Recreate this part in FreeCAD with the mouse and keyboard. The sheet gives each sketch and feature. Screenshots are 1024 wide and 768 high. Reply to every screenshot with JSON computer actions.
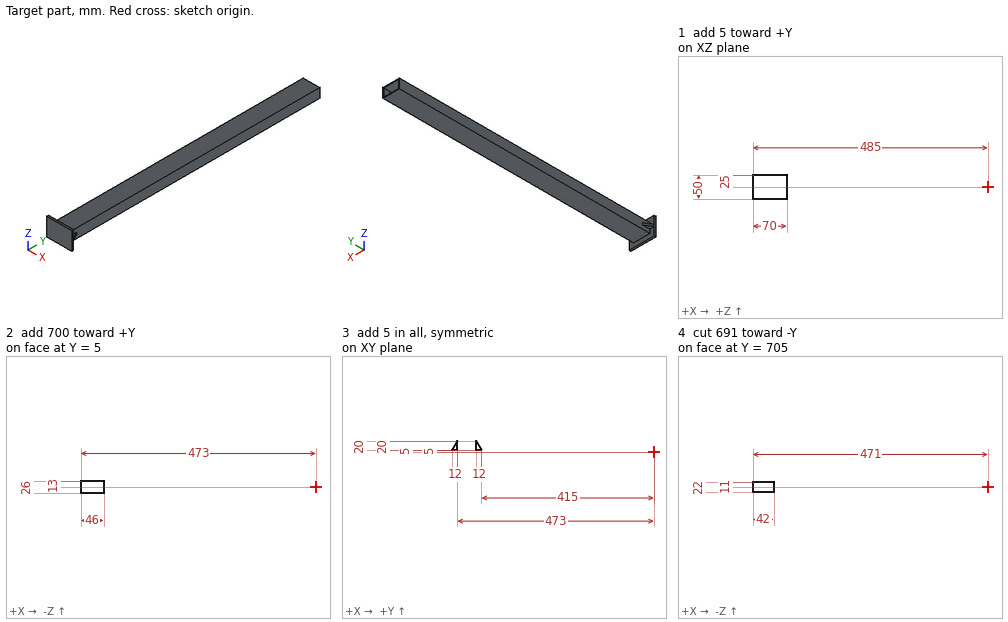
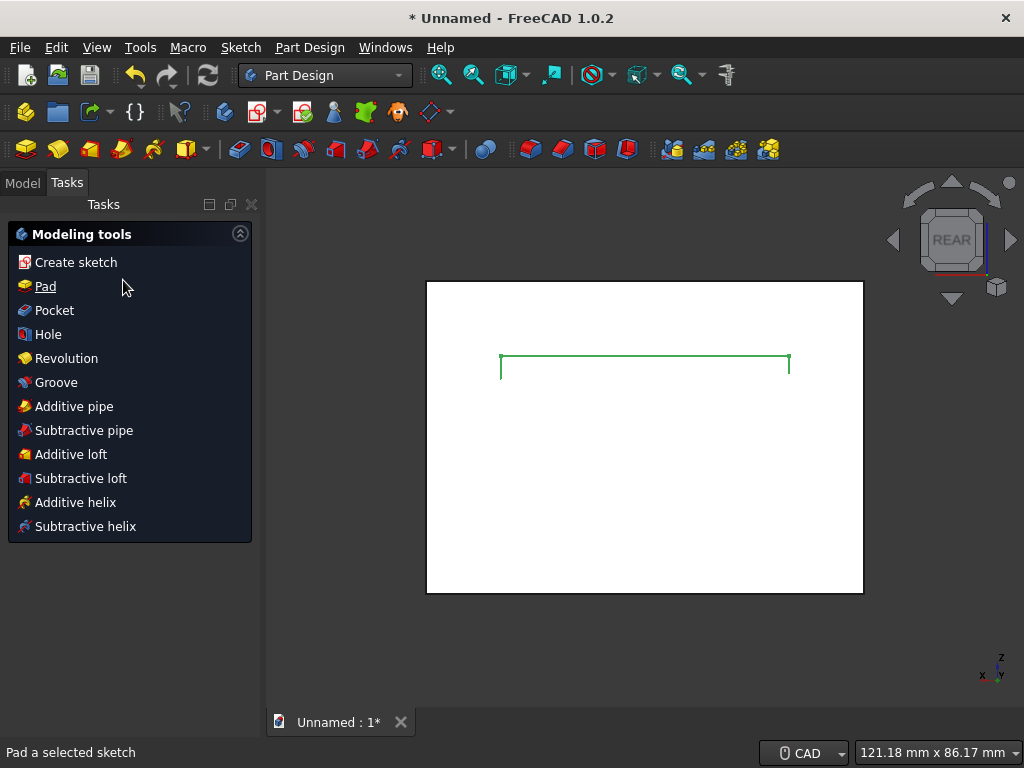
{"action": "left_click", "coordinate": [26, 150]}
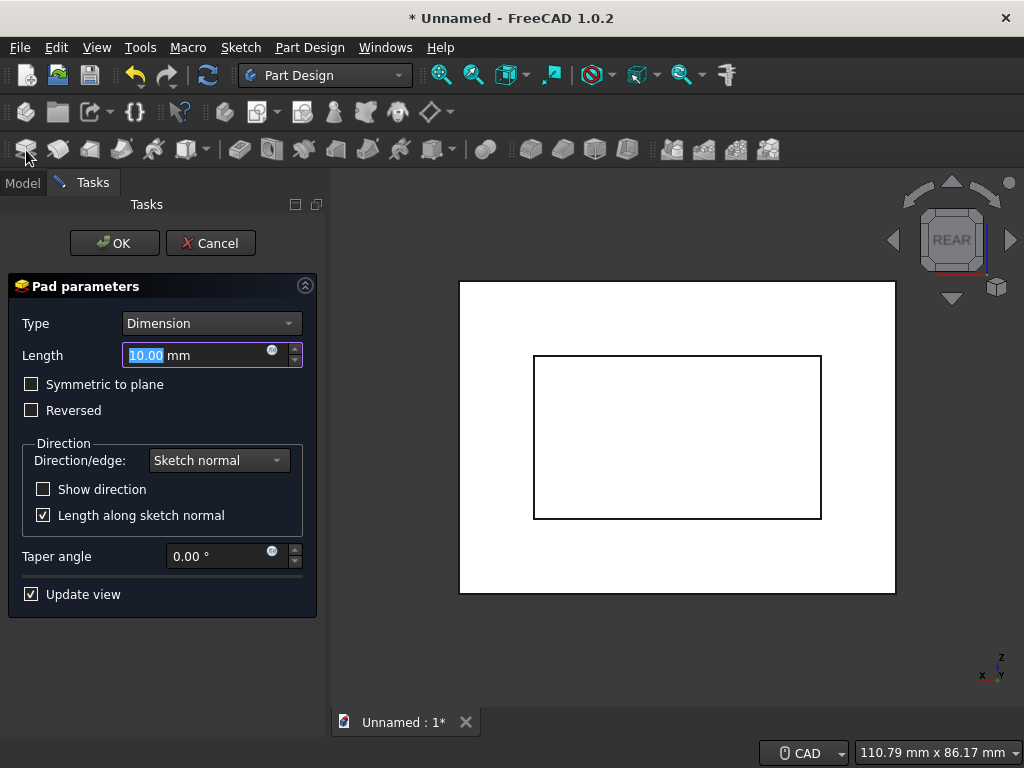
{"action": "type", "text": "700"}
{"action": "key", "text": "Tab"}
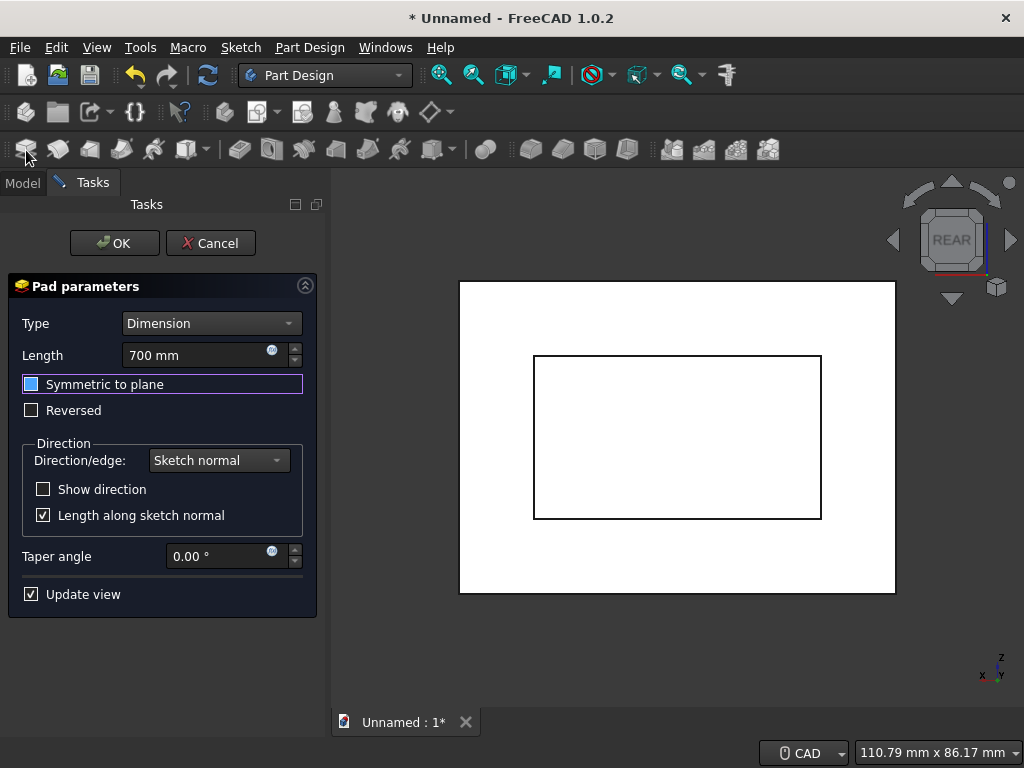
{"action": "left_click", "coordinate": [115, 243]}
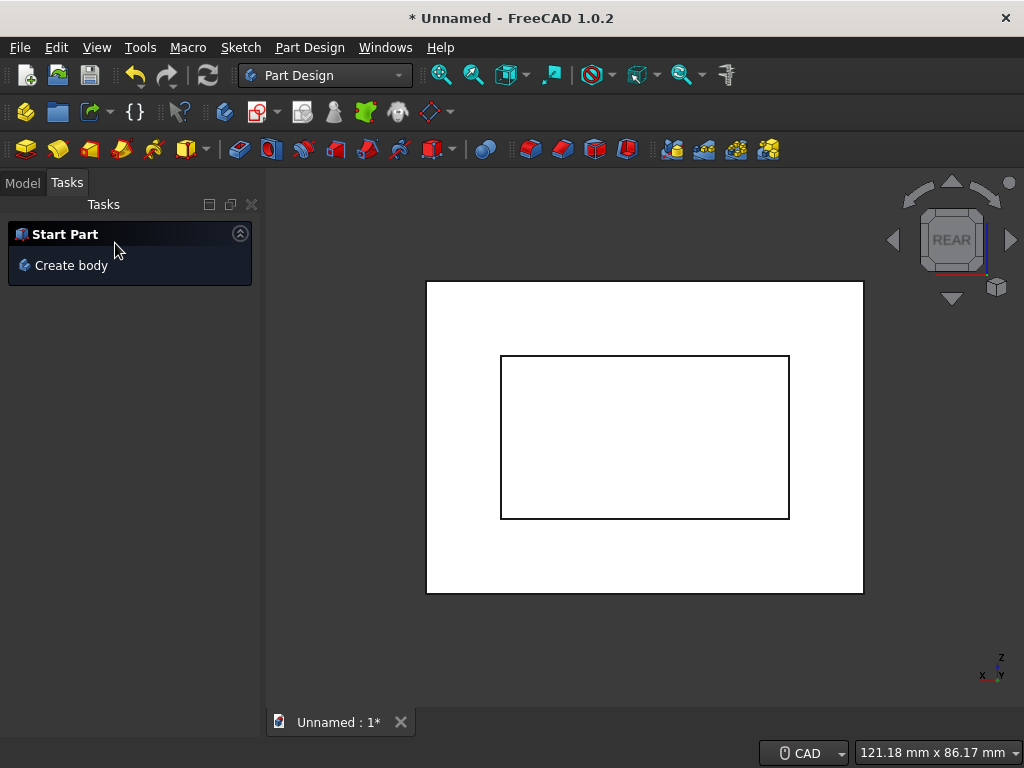
{"action": "left_click", "coordinate": [258, 112]}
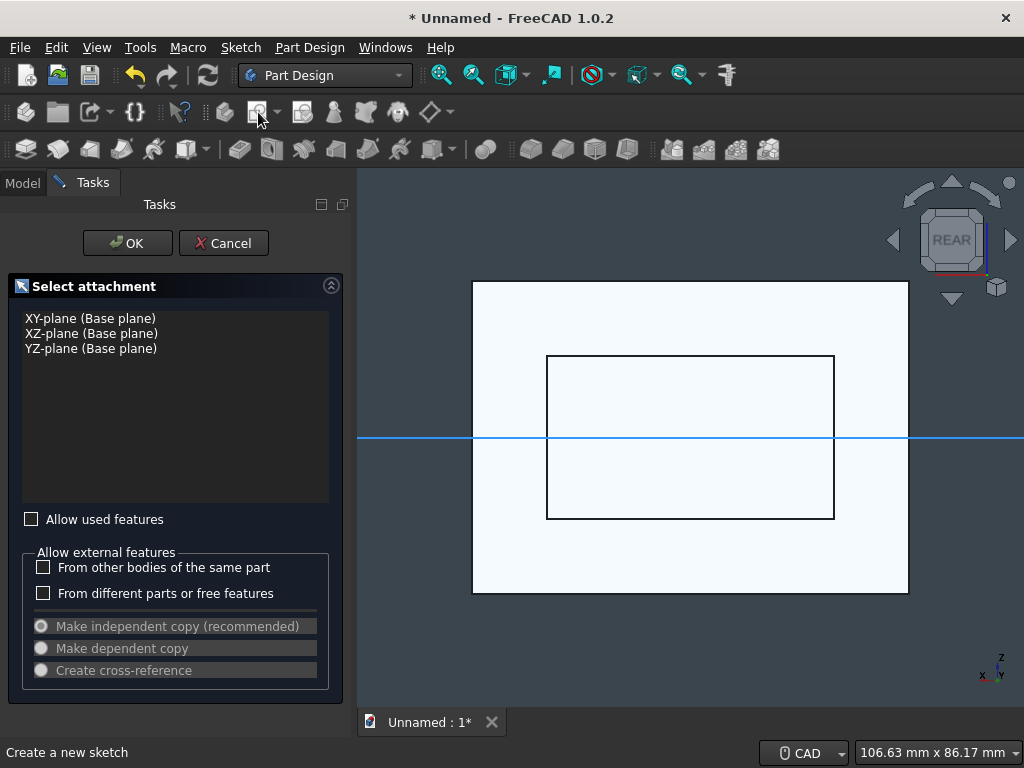
{"action": "left_click", "coordinate": [82, 318]}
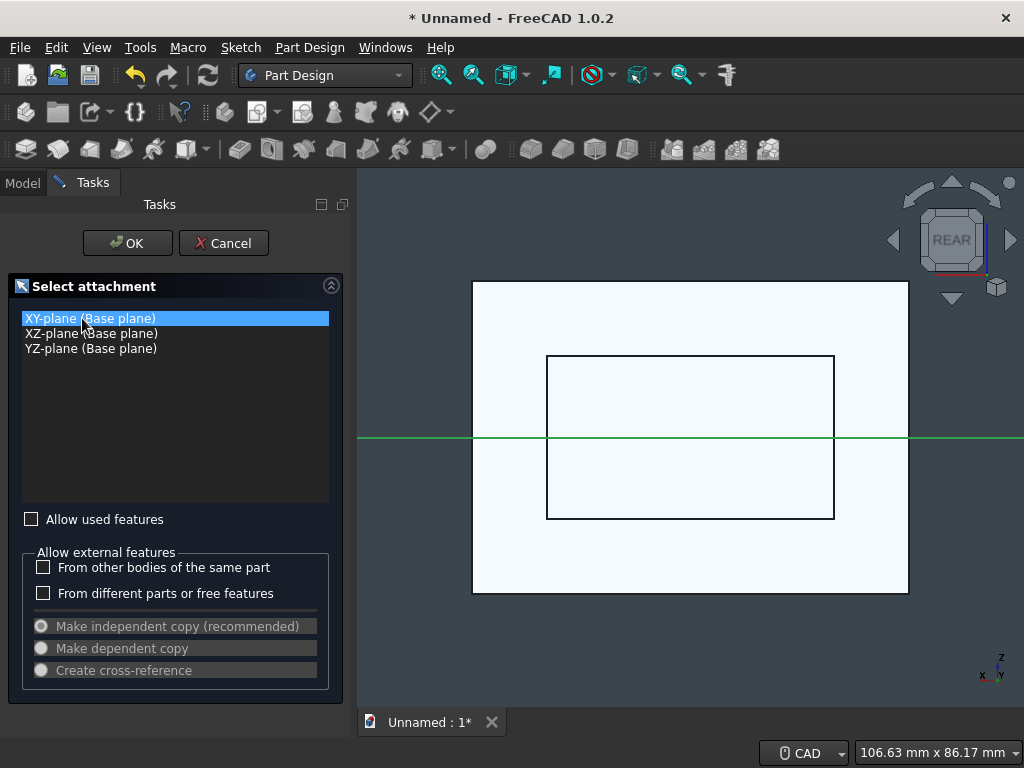
{"action": "left_click", "coordinate": [128, 243]}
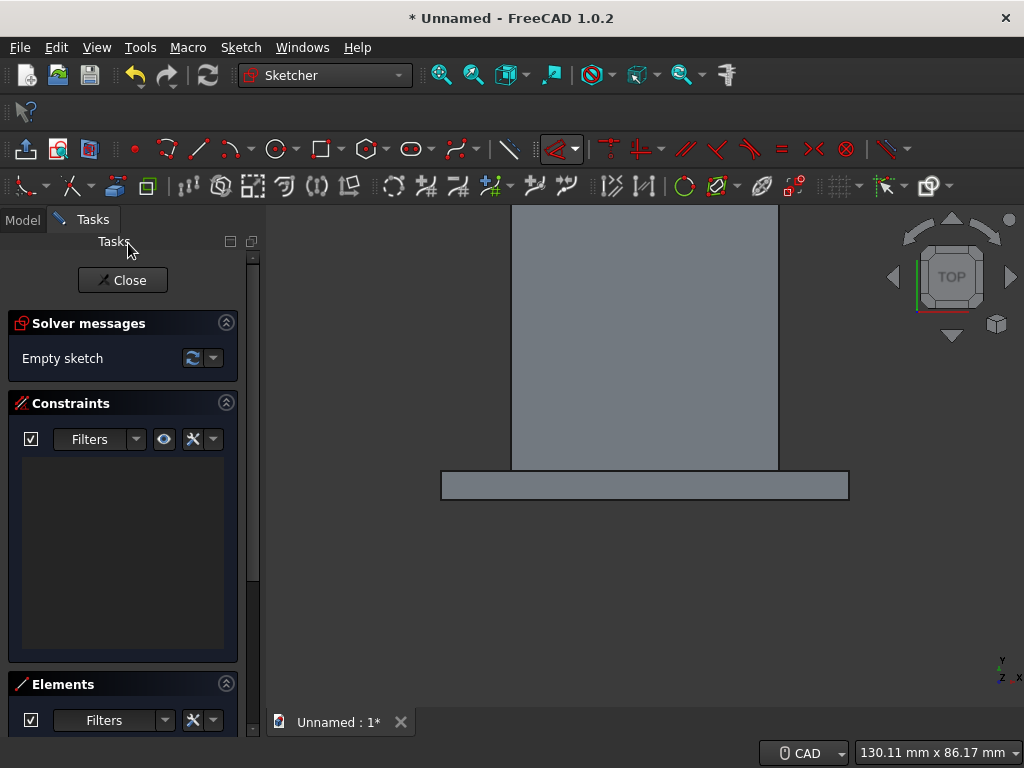
{"action": "left_click", "coordinate": [90, 150]}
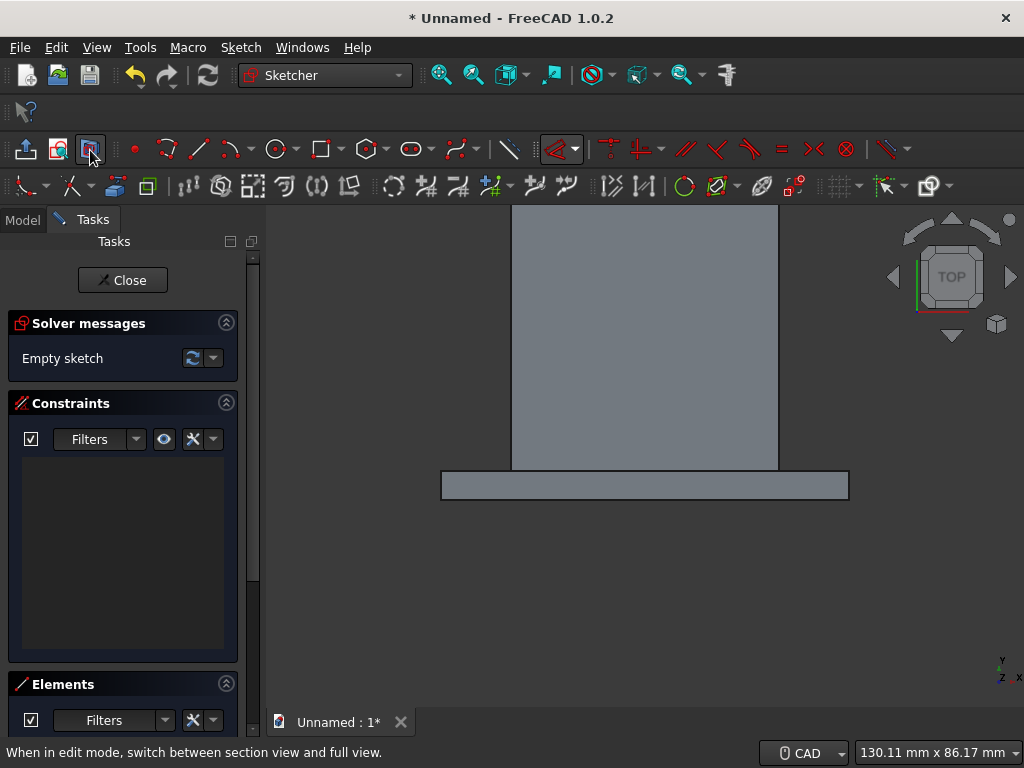
{"action": "scroll", "coordinate": [294, 653], "scroll_direction": "down", "scroll_amount": 1}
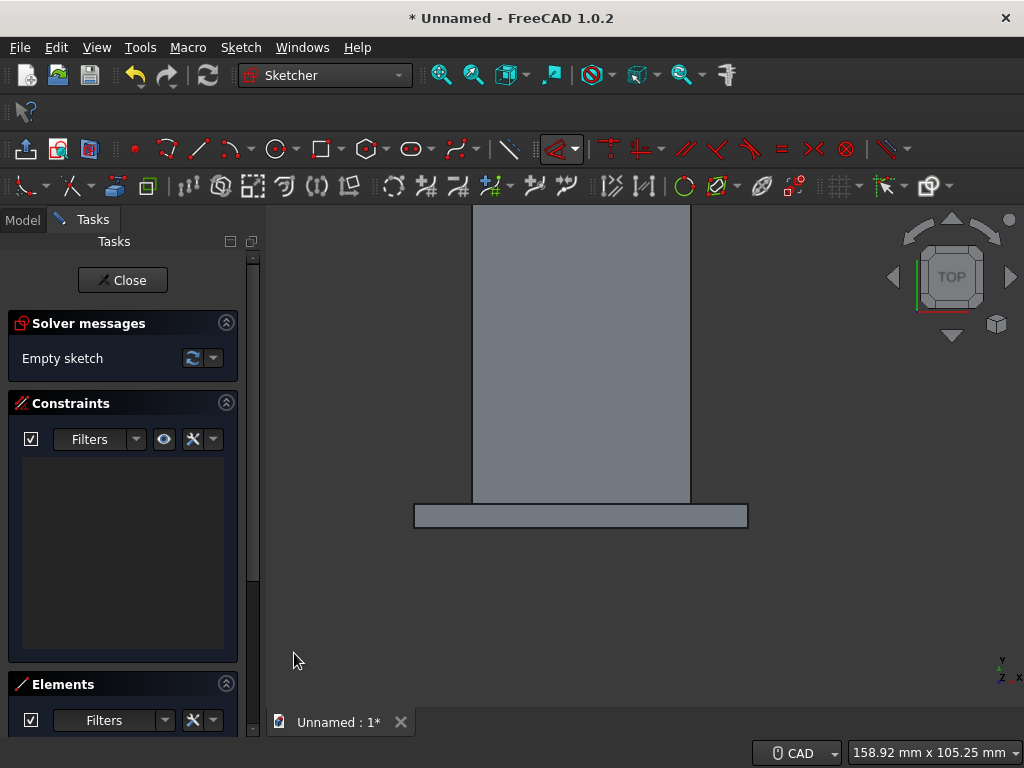
{"action": "left_click", "coordinate": [168, 150]}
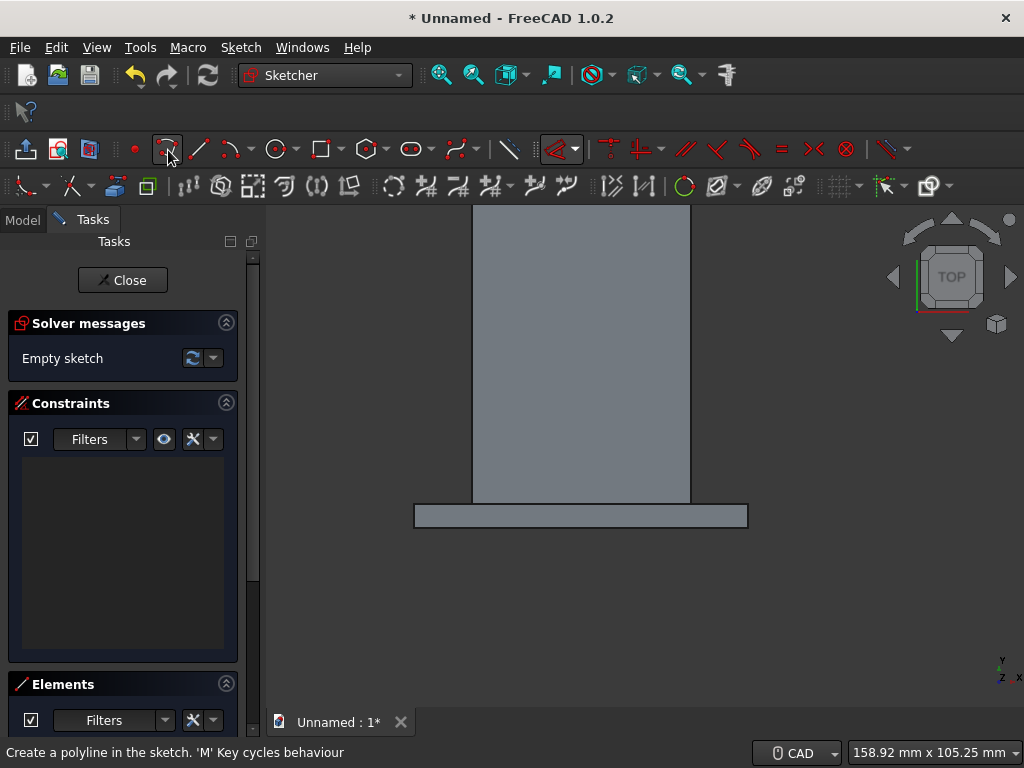
{"action": "left_click", "coordinate": [472, 504]}
{"action": "left_click", "coordinate": [472, 408]}
{"action": "left_click", "coordinate": [414, 504]}
{"action": "left_click", "coordinate": [472, 505]}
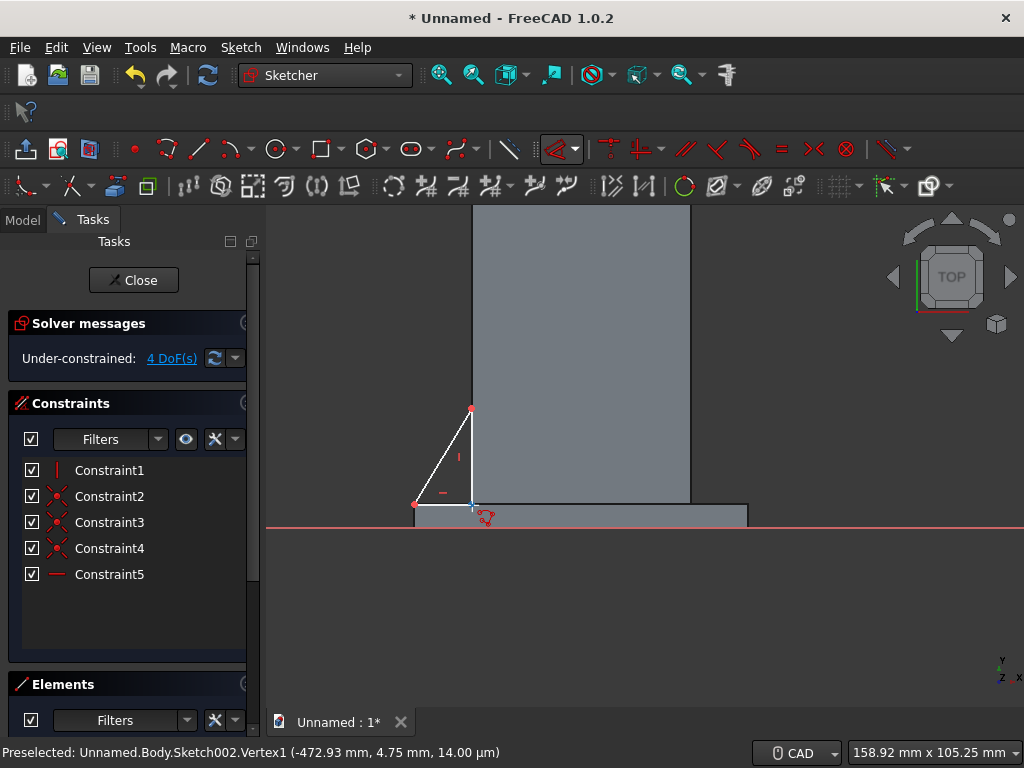
{"action": "left_click", "coordinate": [748, 504]}
{"action": "left_click", "coordinate": [691, 408]}
{"action": "left_click", "coordinate": [691, 504]}
{"action": "left_click", "coordinate": [748, 505]}
{"action": "key", "text": "Escape"}
{"action": "key", "text": "Escape"}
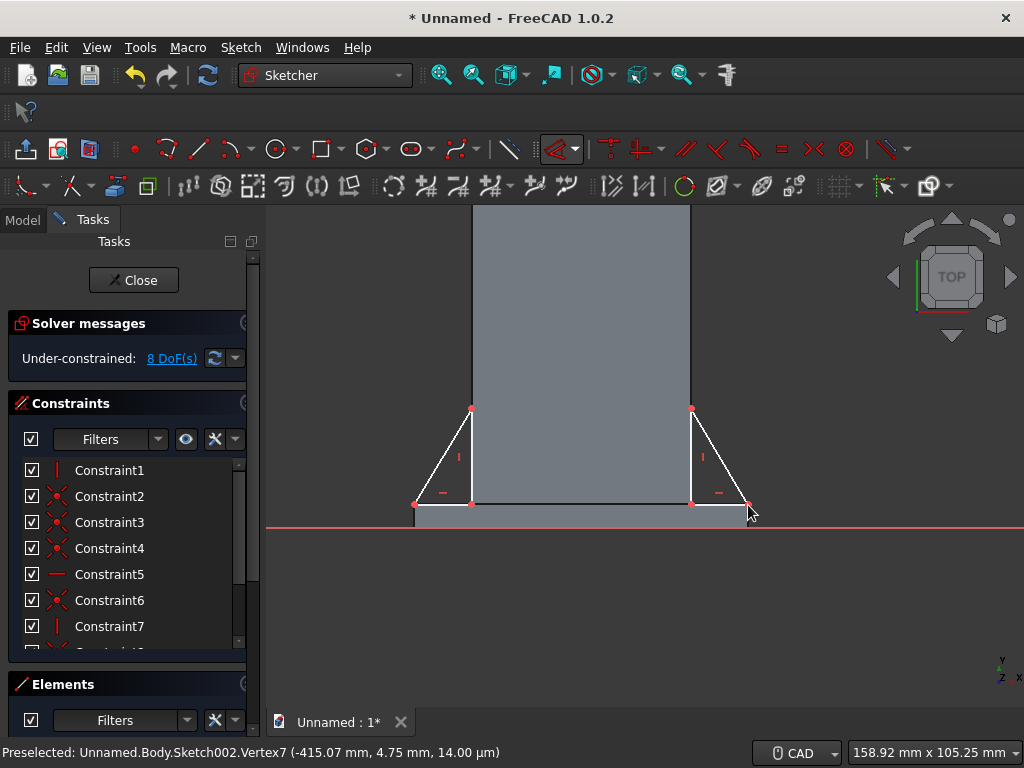
{"action": "left_click", "coordinate": [472, 476]}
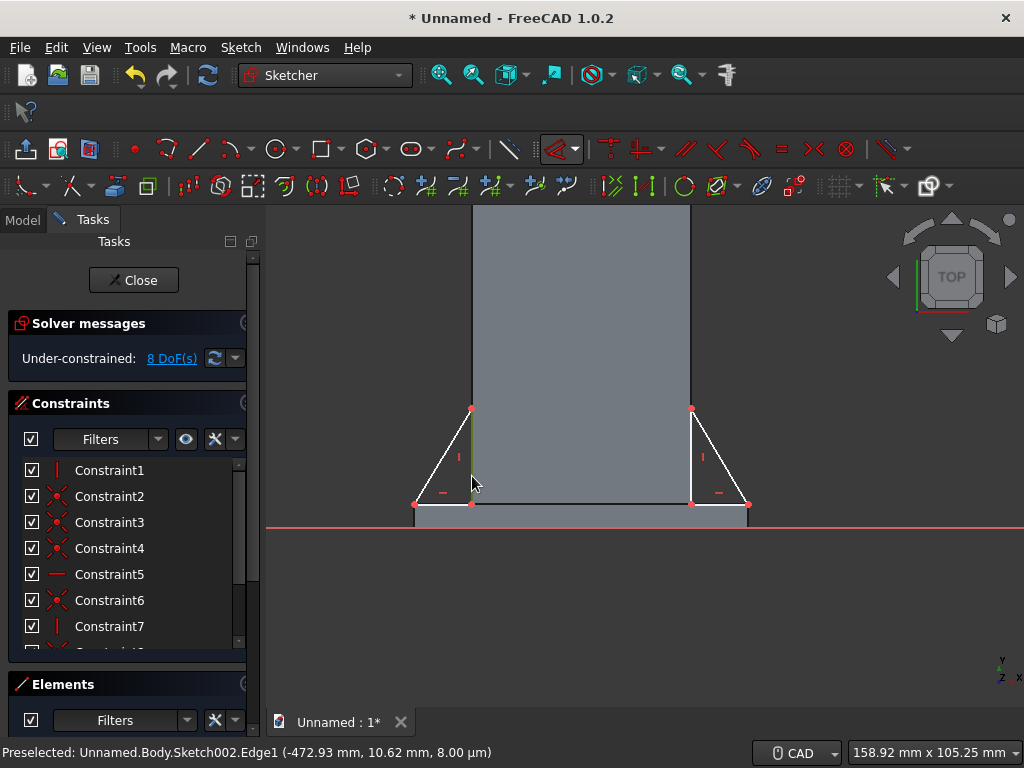
{"action": "key", "text": "i"}